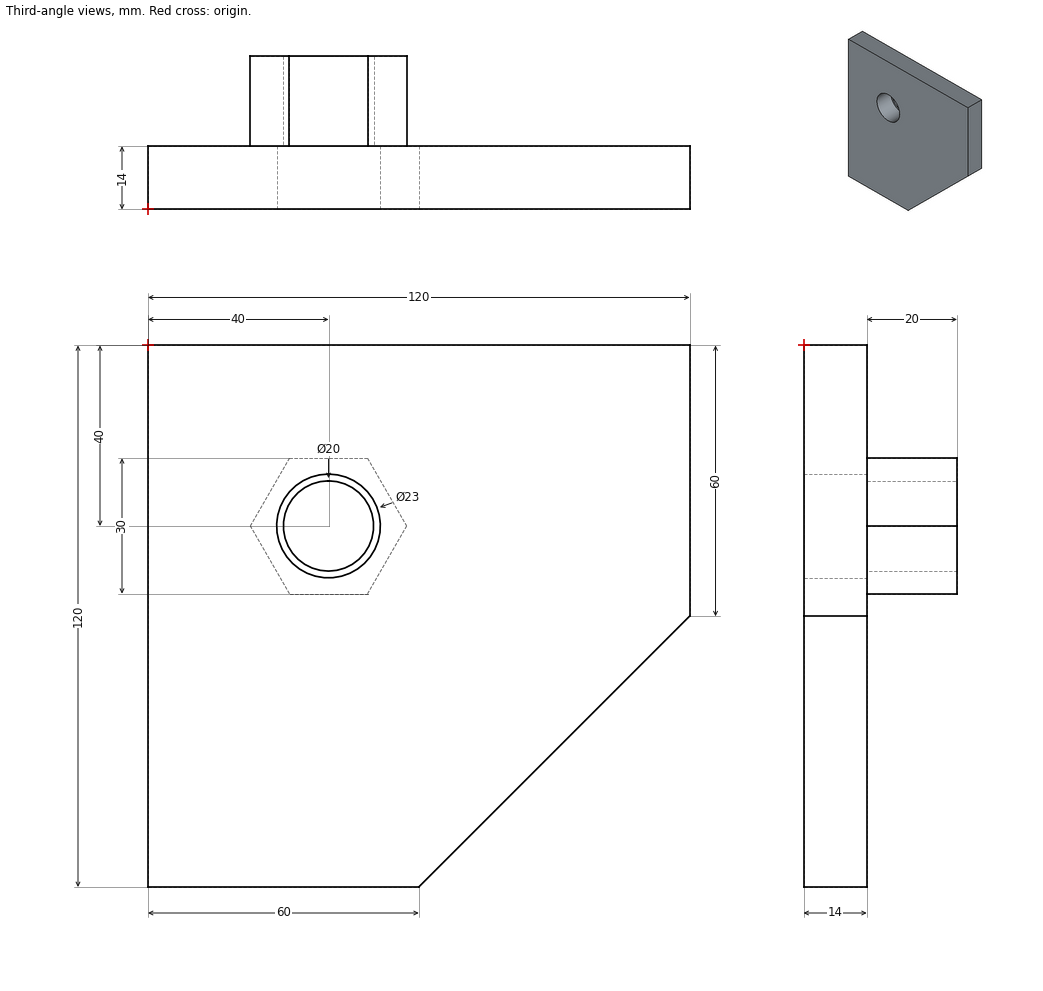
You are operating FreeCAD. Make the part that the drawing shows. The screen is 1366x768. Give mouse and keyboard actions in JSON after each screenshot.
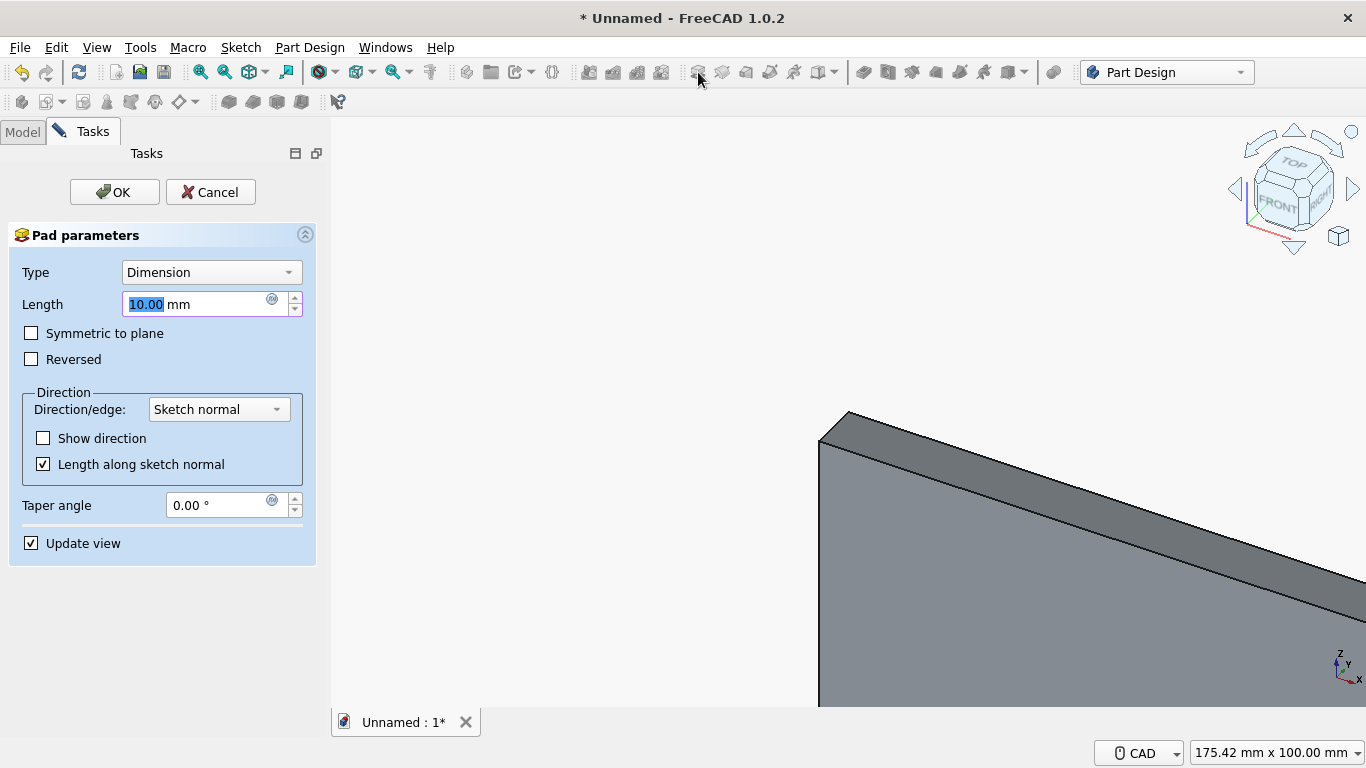
{"action": "type", "text": "14"}
{"action": "key", "text": "Tab"}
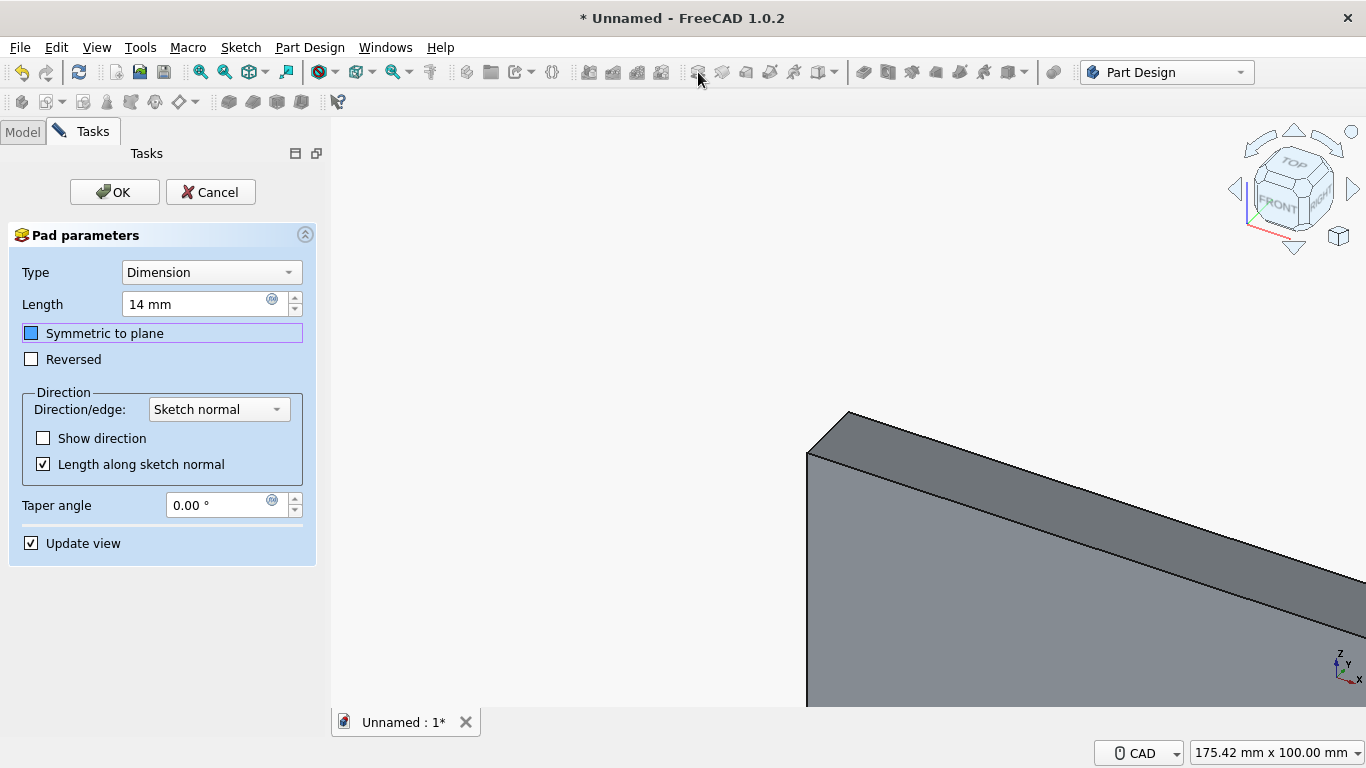
{"action": "left_click", "coordinate": [30, 359]}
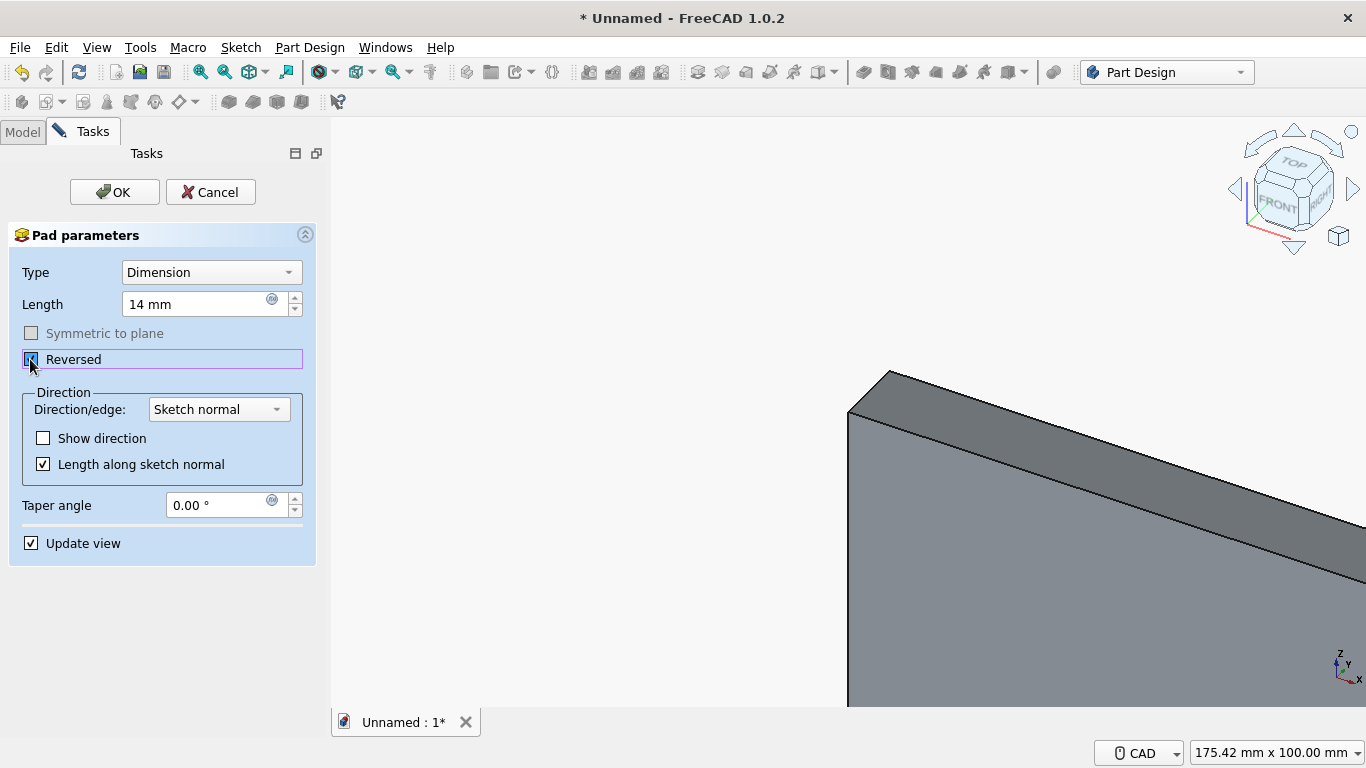
{"action": "left_click", "coordinate": [115, 192]}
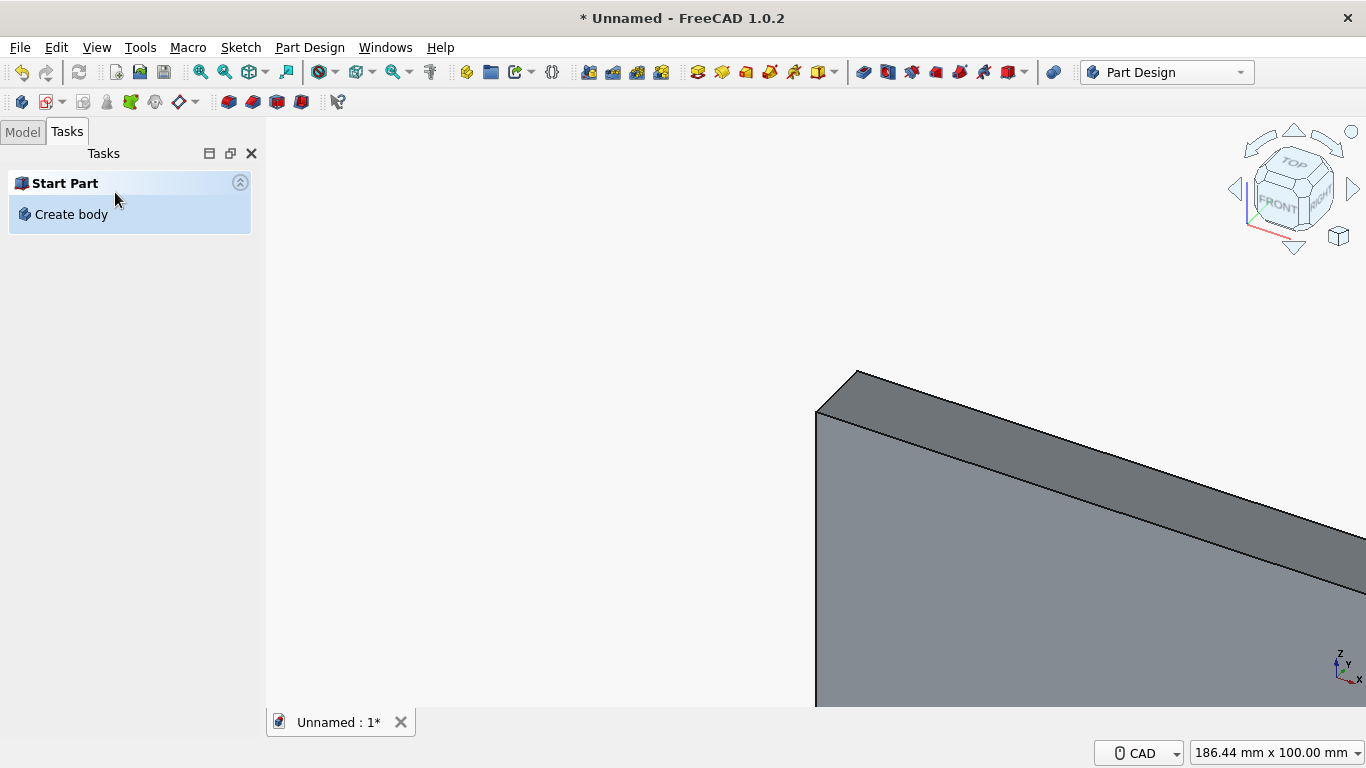
{"action": "left_click", "coordinate": [202, 72]}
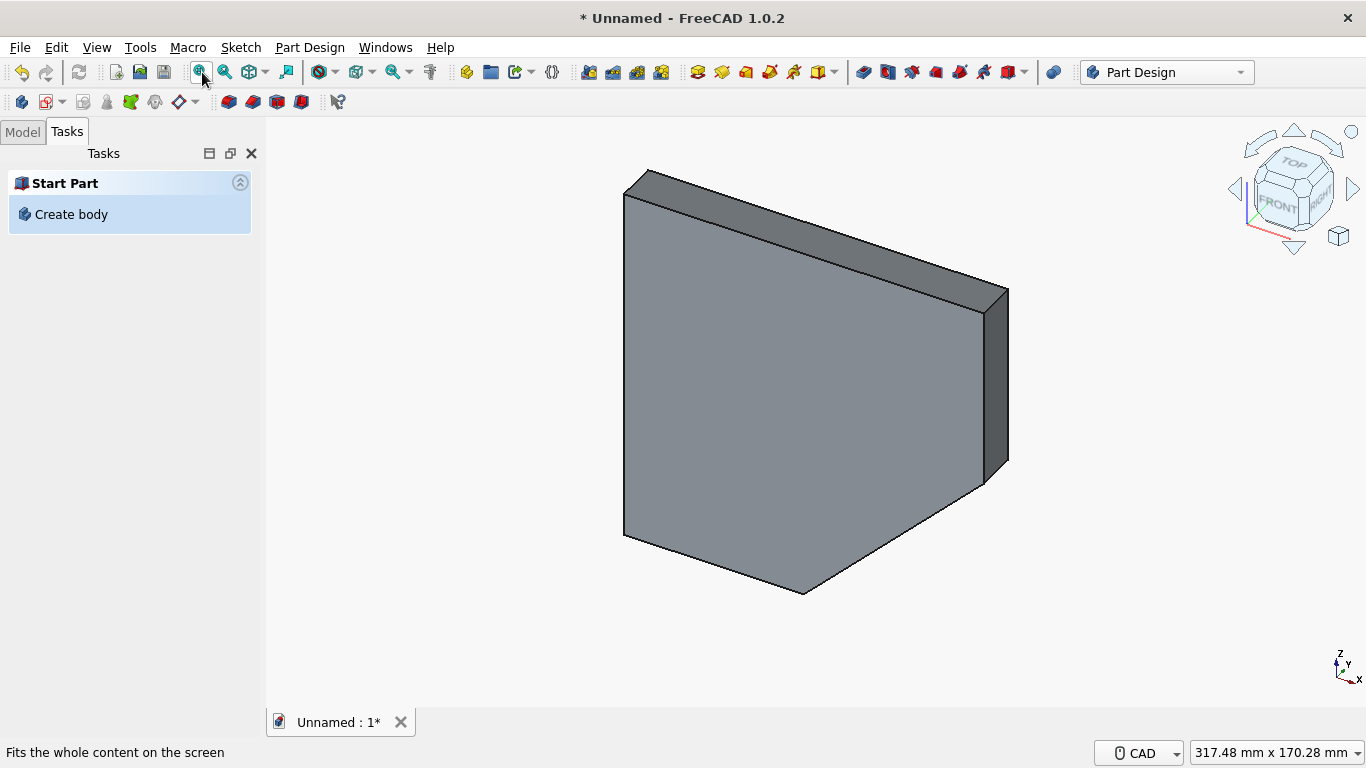
{"action": "key", "text": "4"}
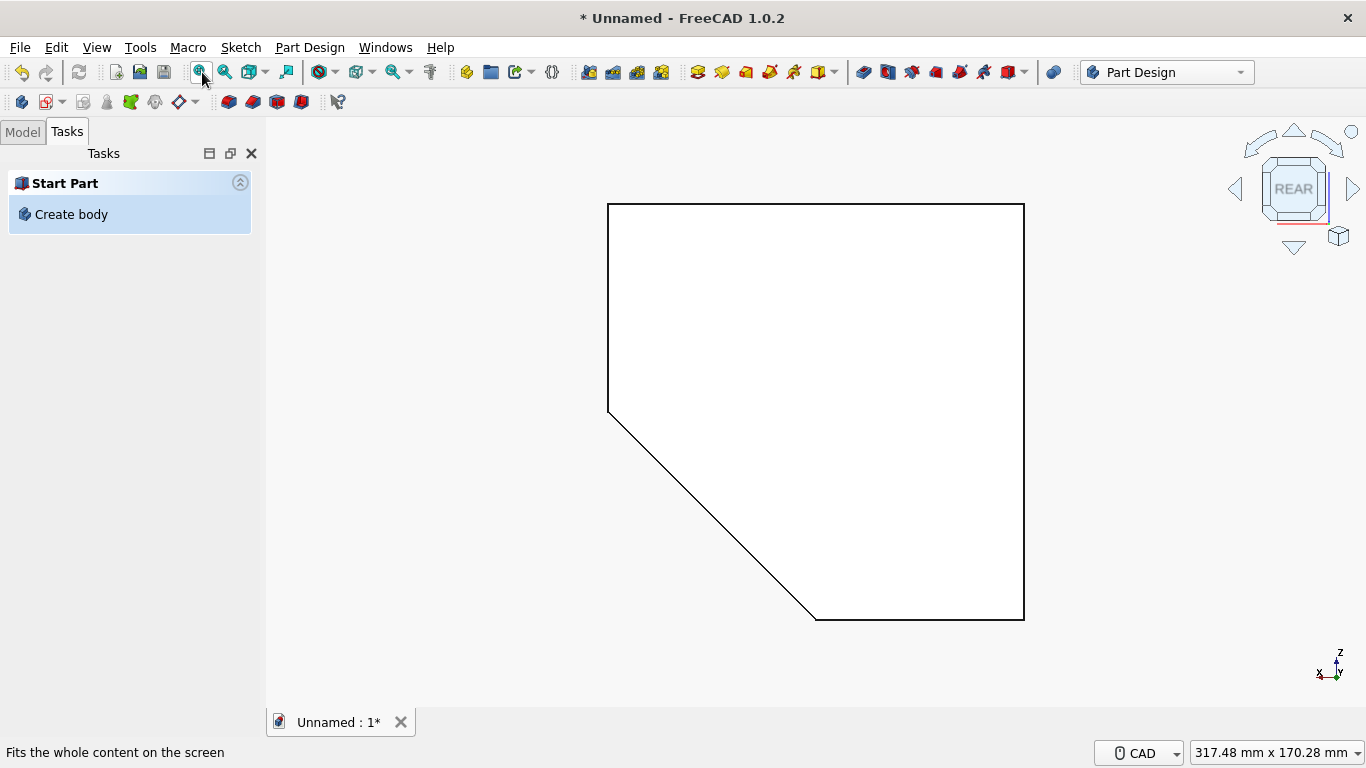
{"action": "left_click", "coordinate": [816, 352]}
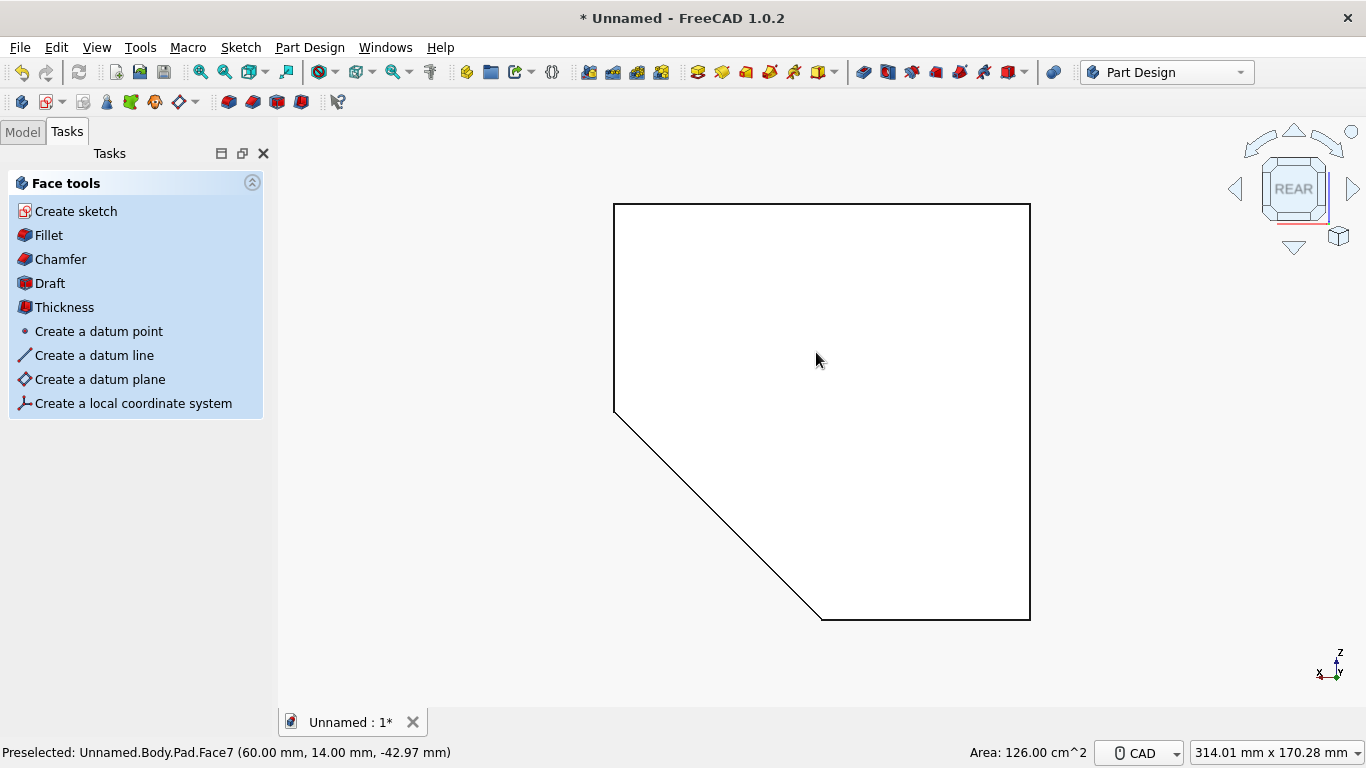
{"action": "left_click", "coordinate": [46, 102]}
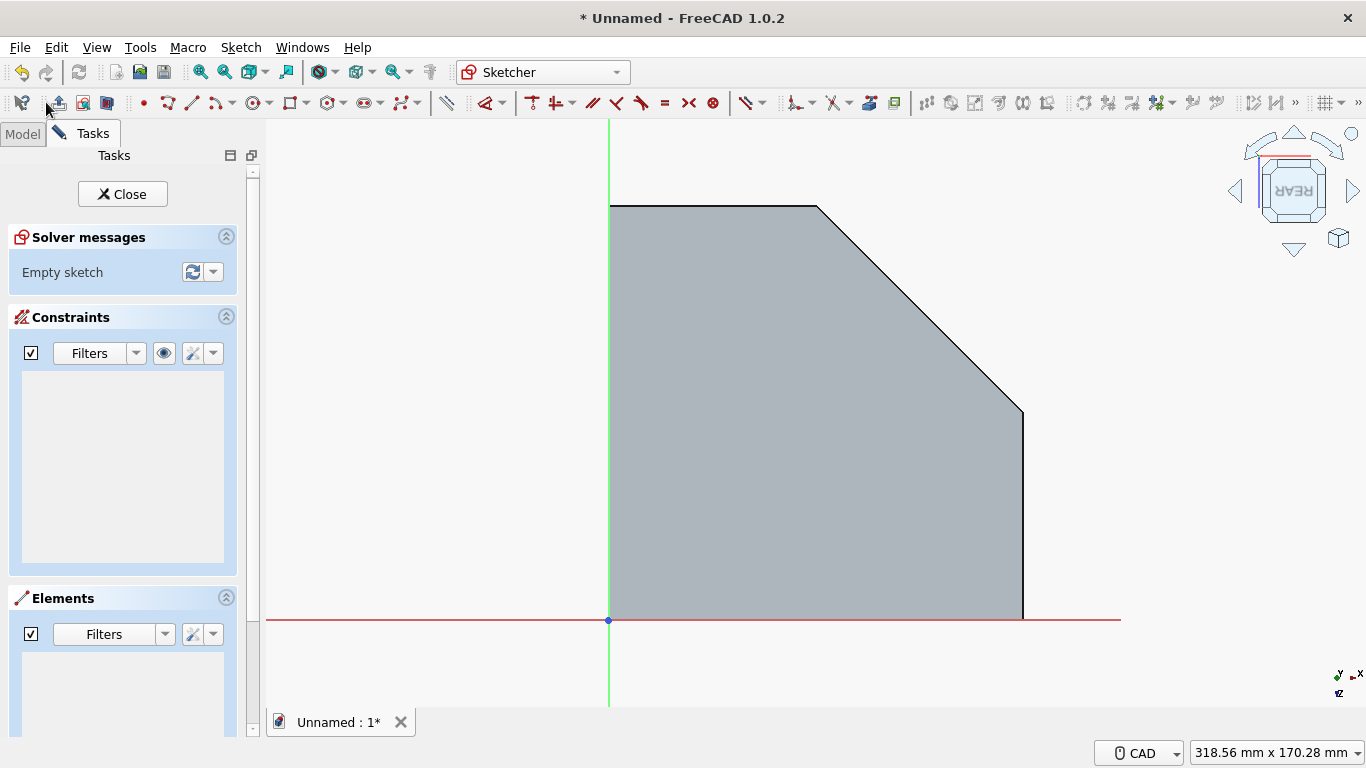
{"action": "scroll", "coordinate": [657, 628], "scroll_direction": "up", "scroll_amount": 4}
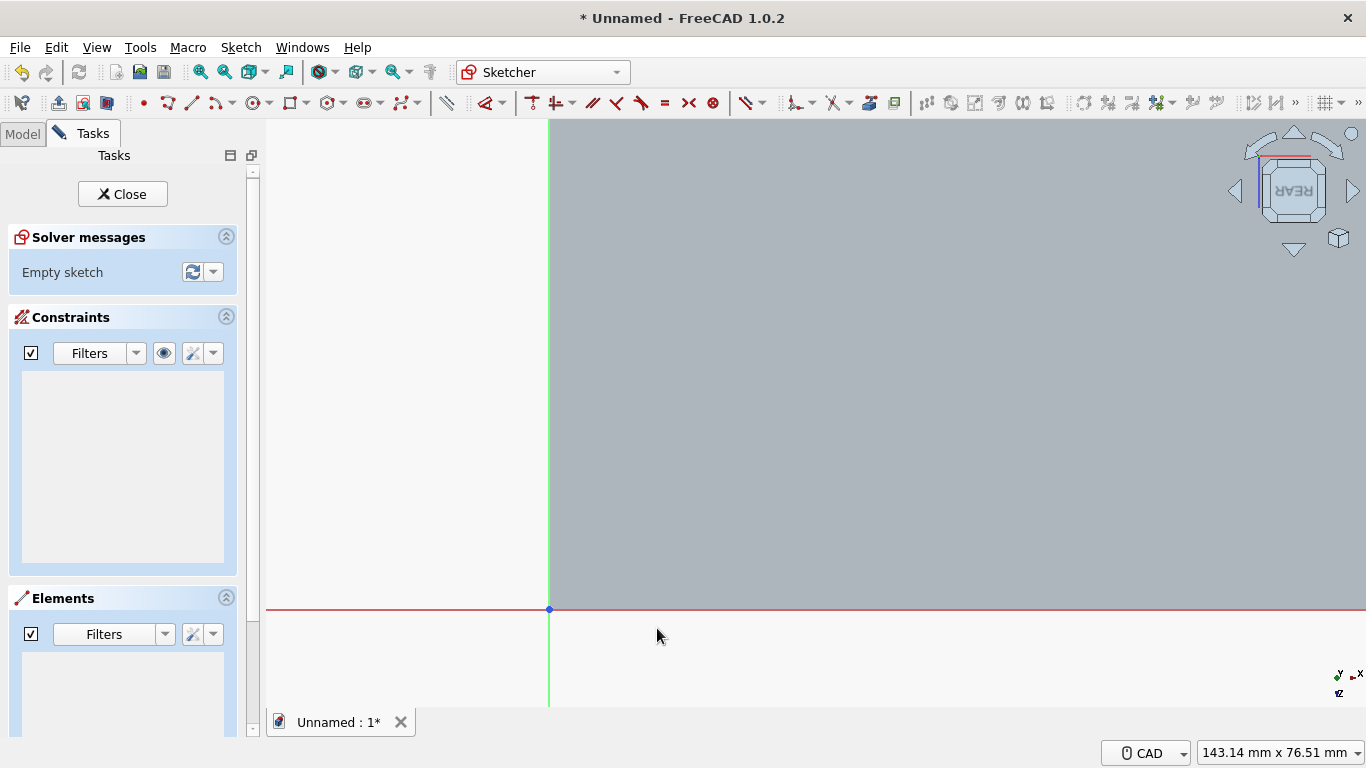
{"action": "left_click", "coordinate": [254, 104]}